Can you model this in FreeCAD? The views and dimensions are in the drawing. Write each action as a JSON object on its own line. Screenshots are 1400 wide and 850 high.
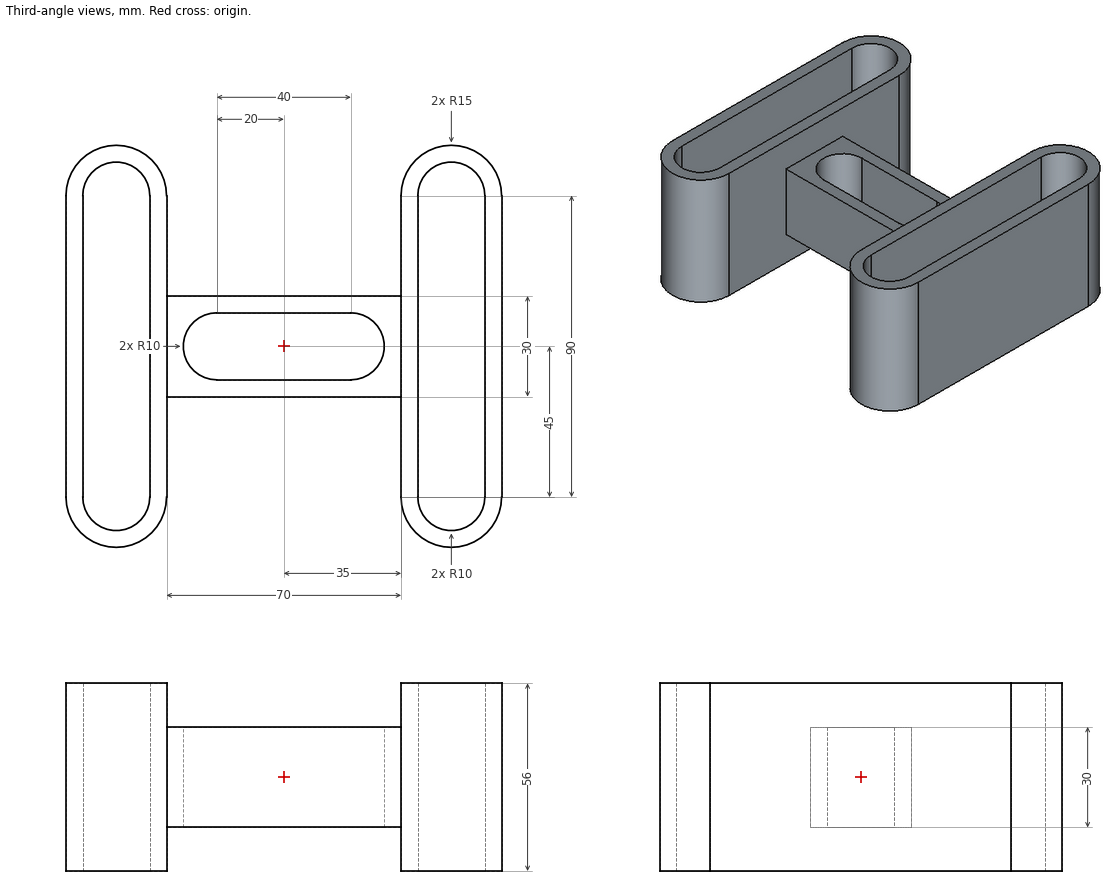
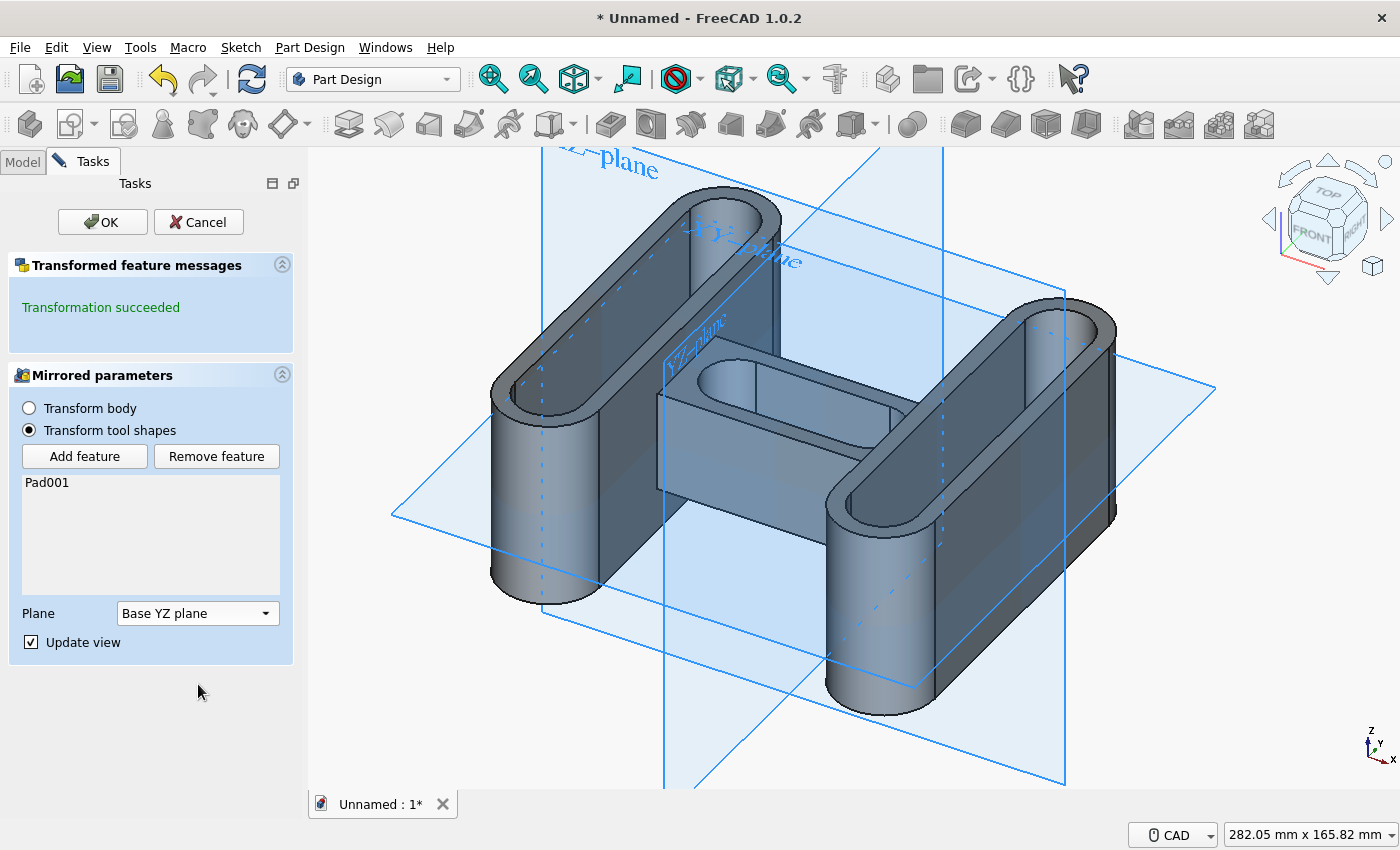
{"action": "left_click", "coordinate": [103, 222]}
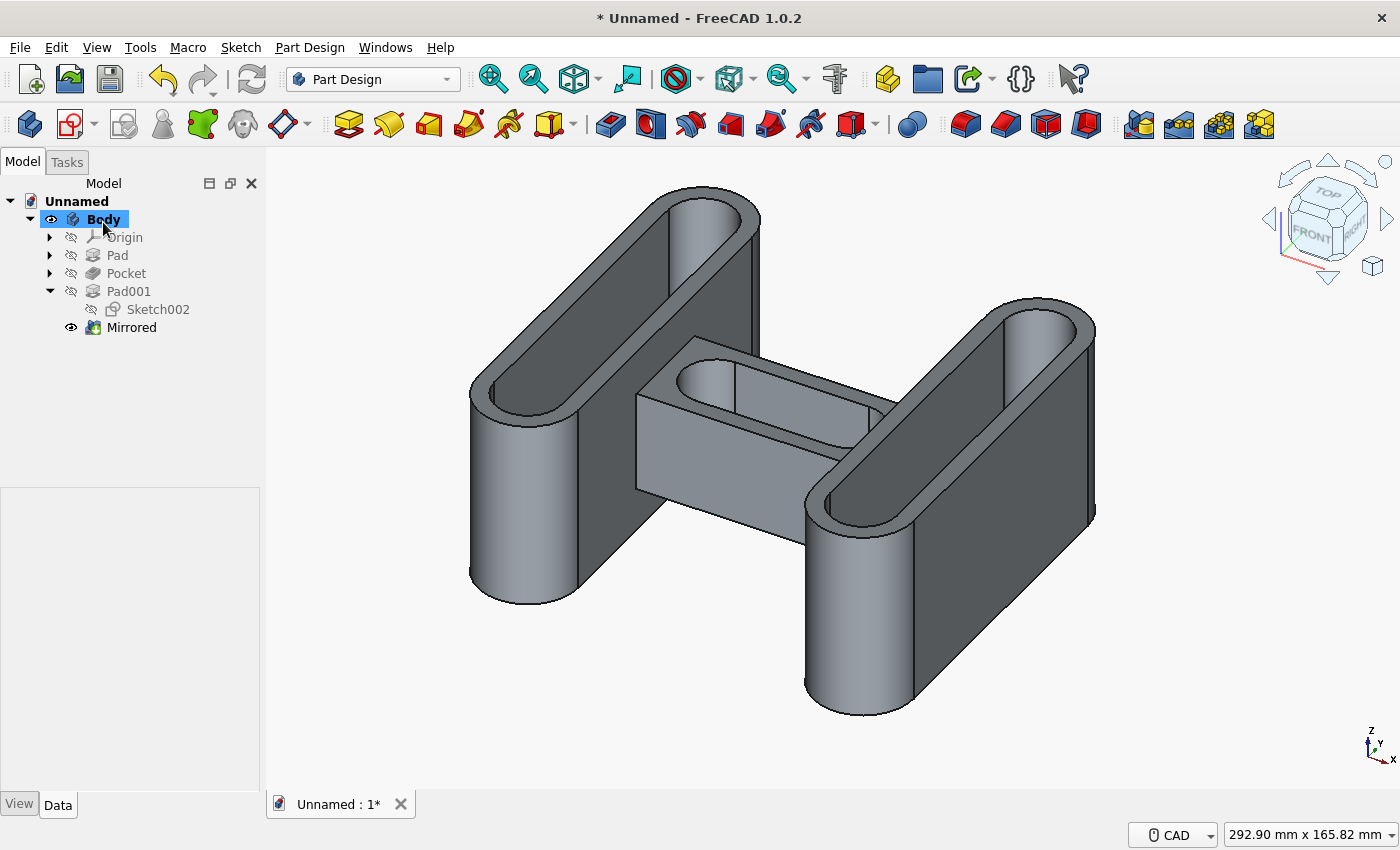
{"action": "key", "text": "0"}